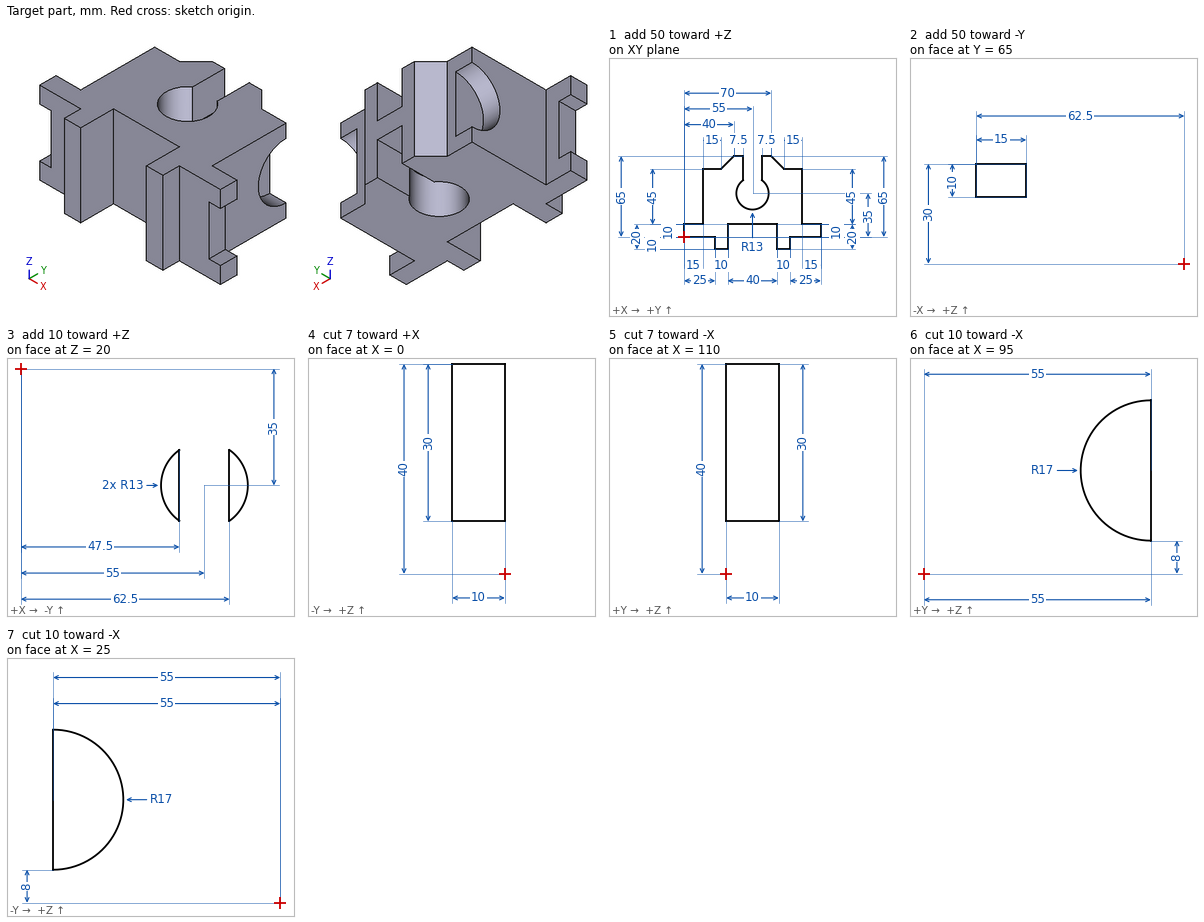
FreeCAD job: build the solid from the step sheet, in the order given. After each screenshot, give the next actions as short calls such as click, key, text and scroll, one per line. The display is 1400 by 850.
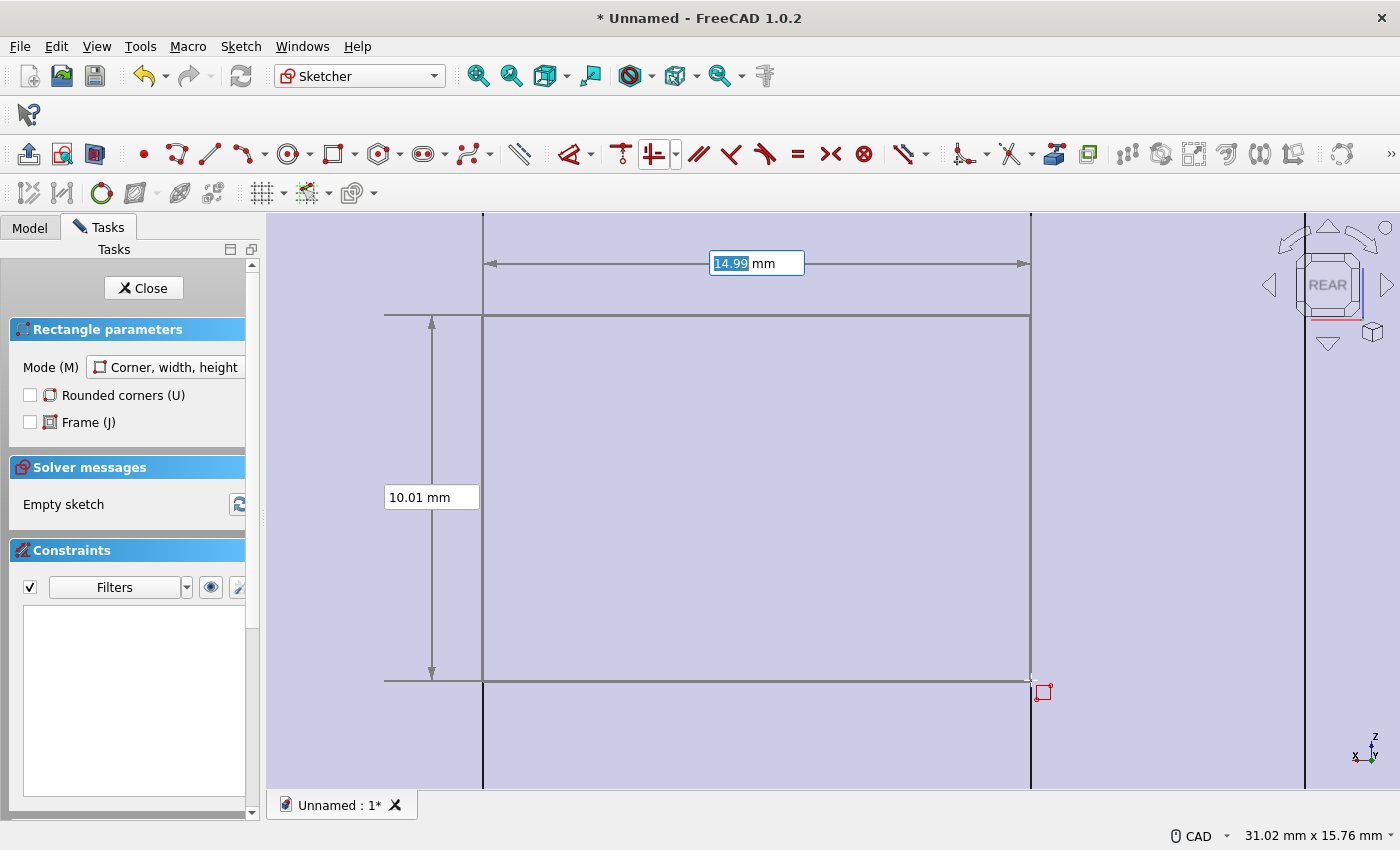
text(15)
key(Tab)
text(10)
key(Return)
key(Escape)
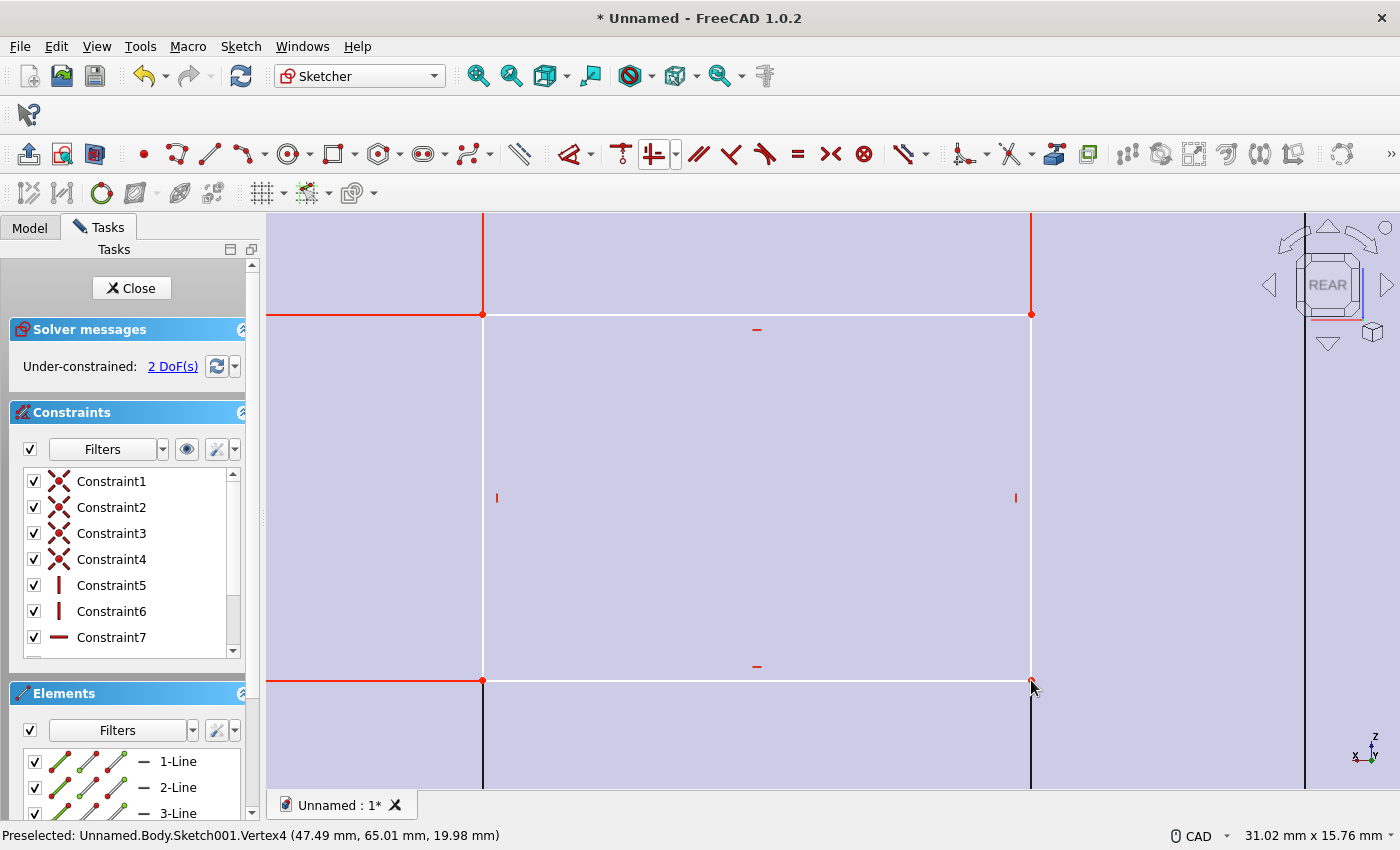
click(568, 154)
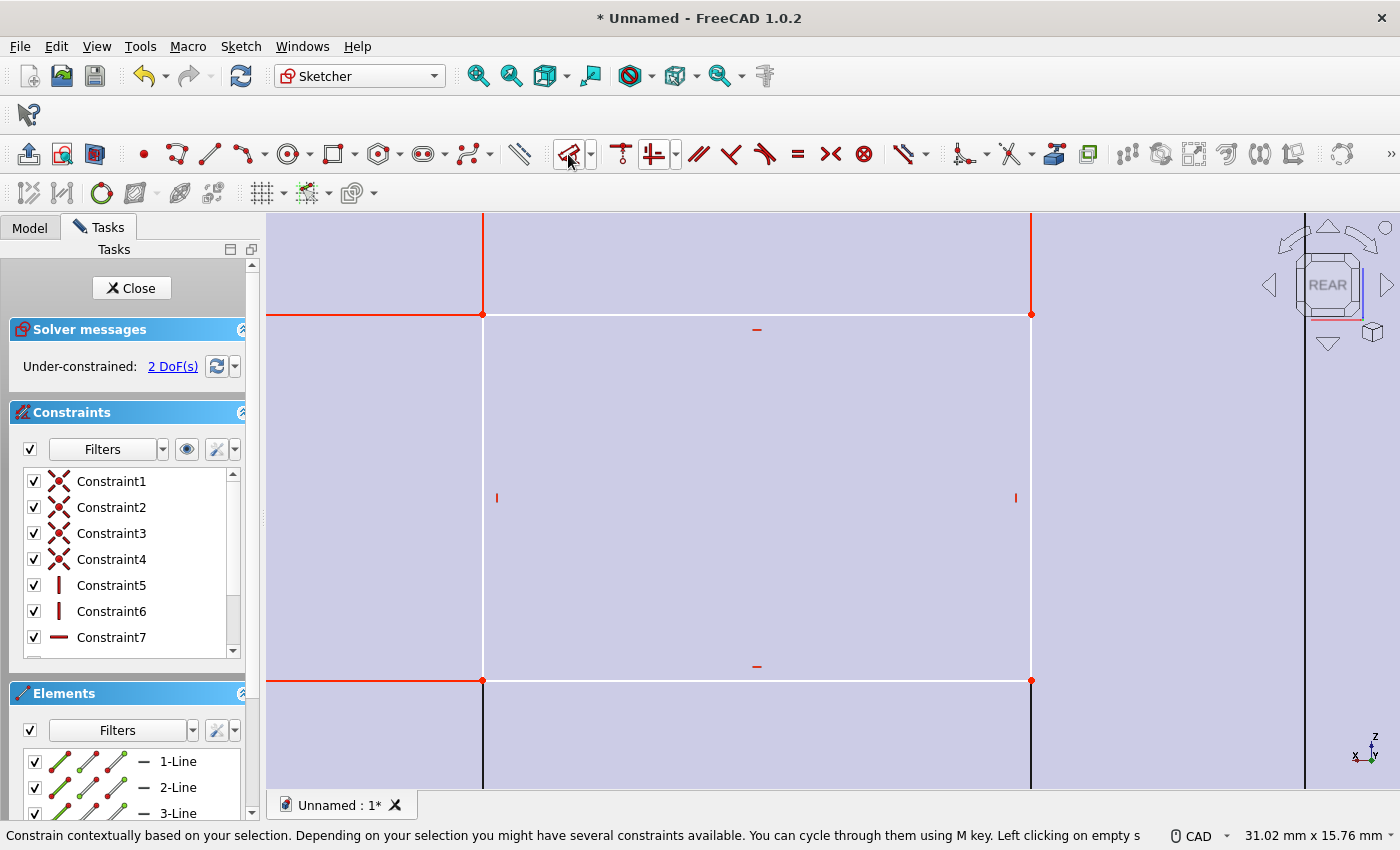
click(483, 315)
click(449, 538)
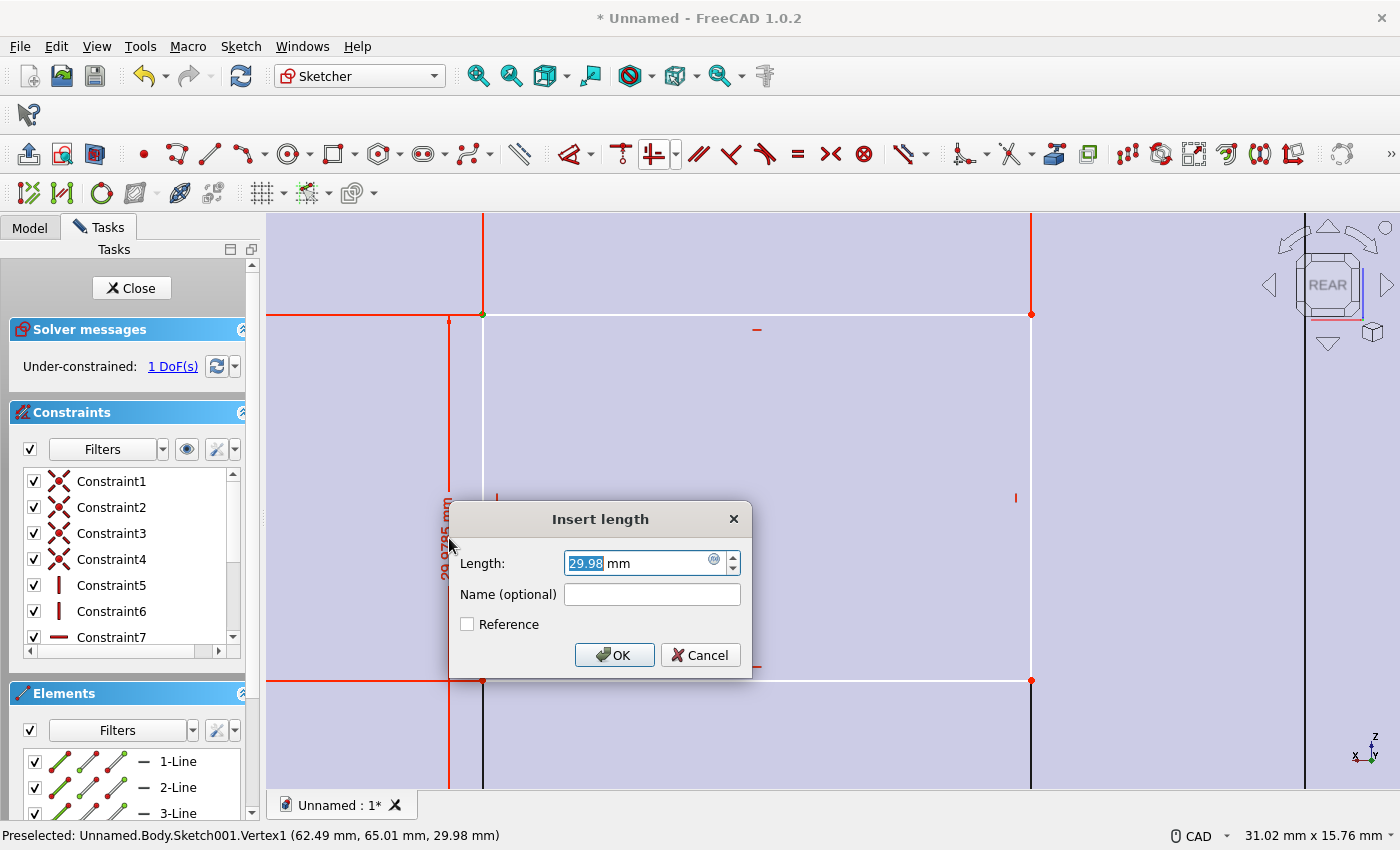
text(30)
key(Return)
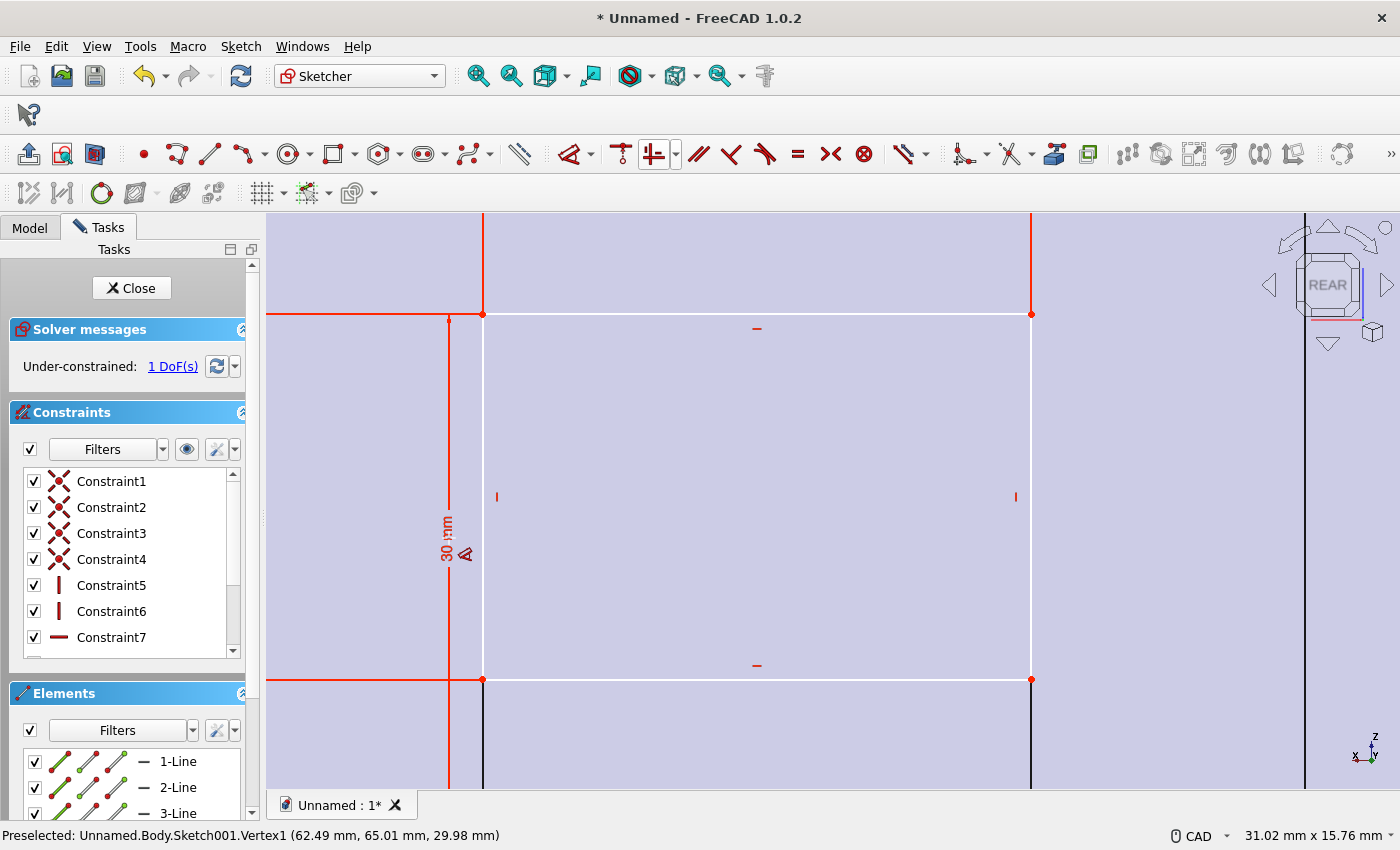
click(483, 314)
click(859, 280)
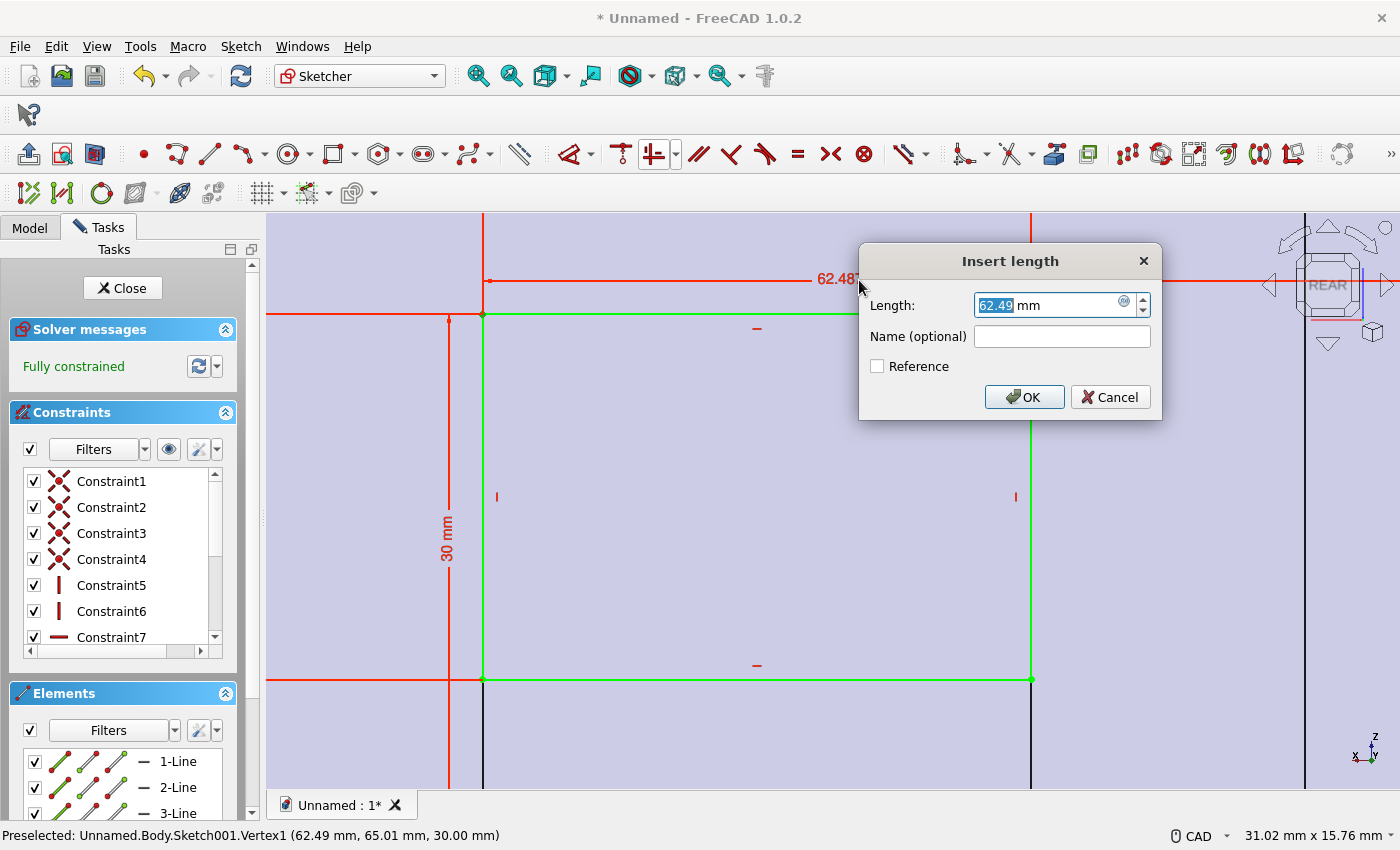
text(62.5)
key(Return)
key(Escape)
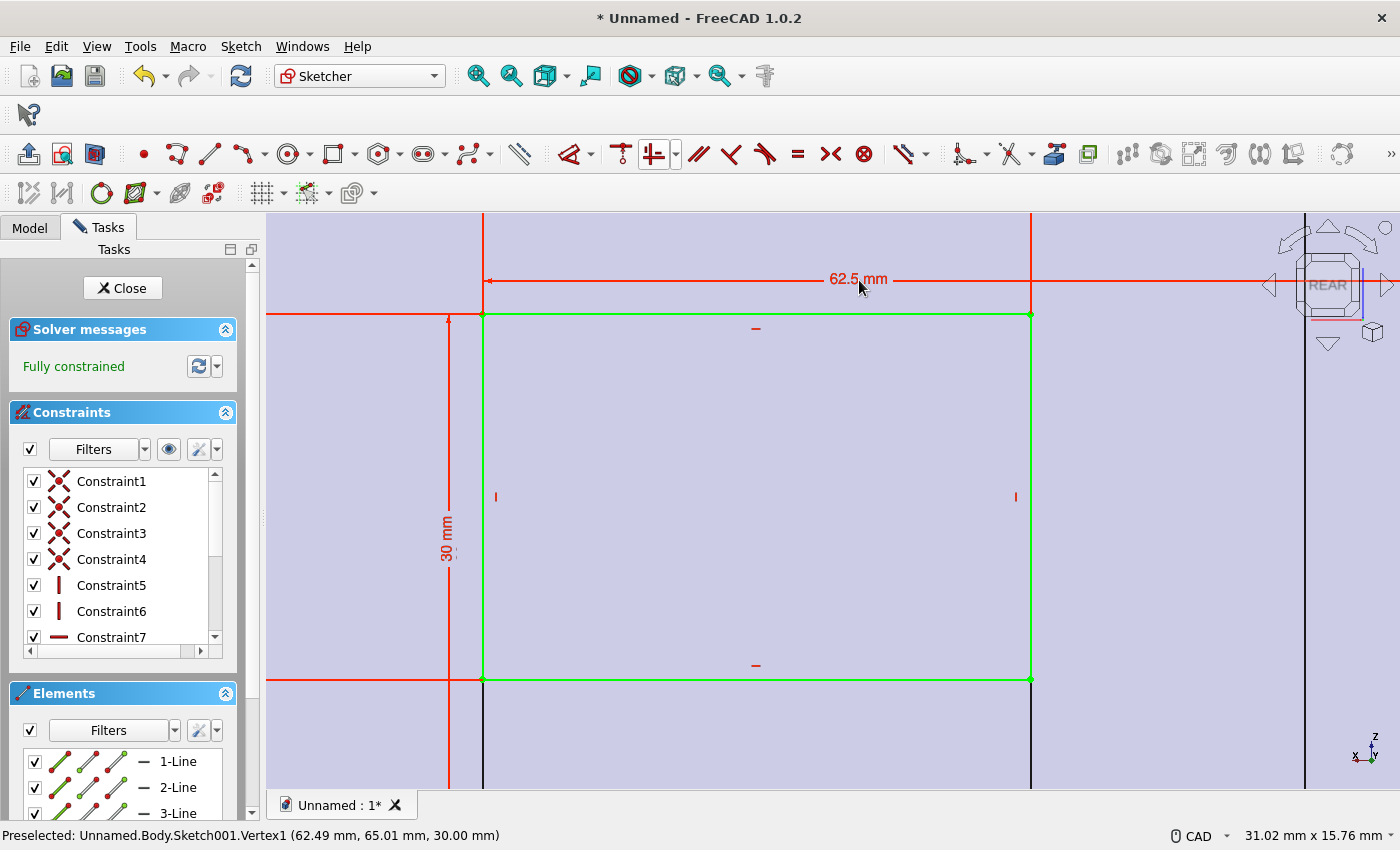
click(123, 288)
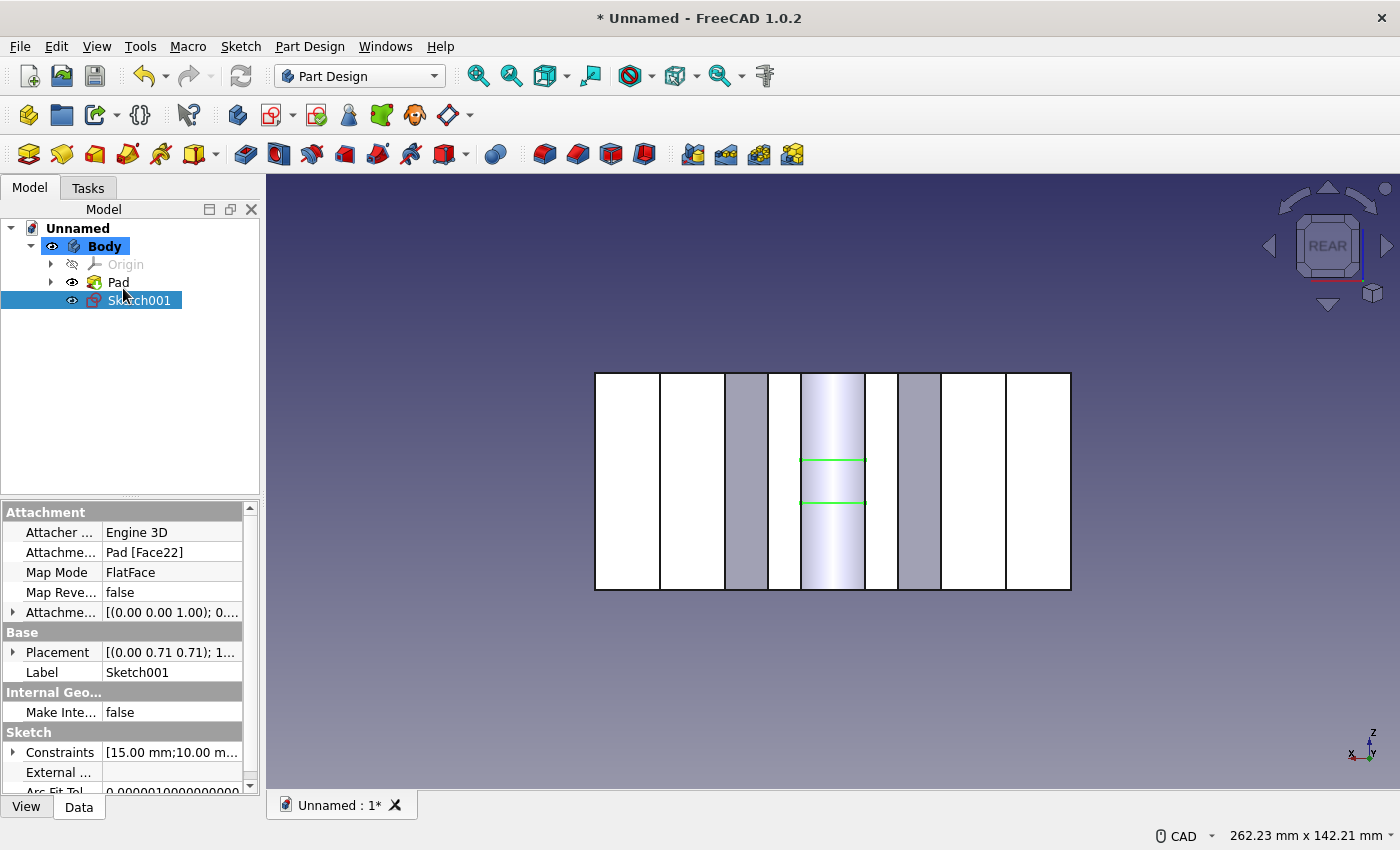
click(29, 154)